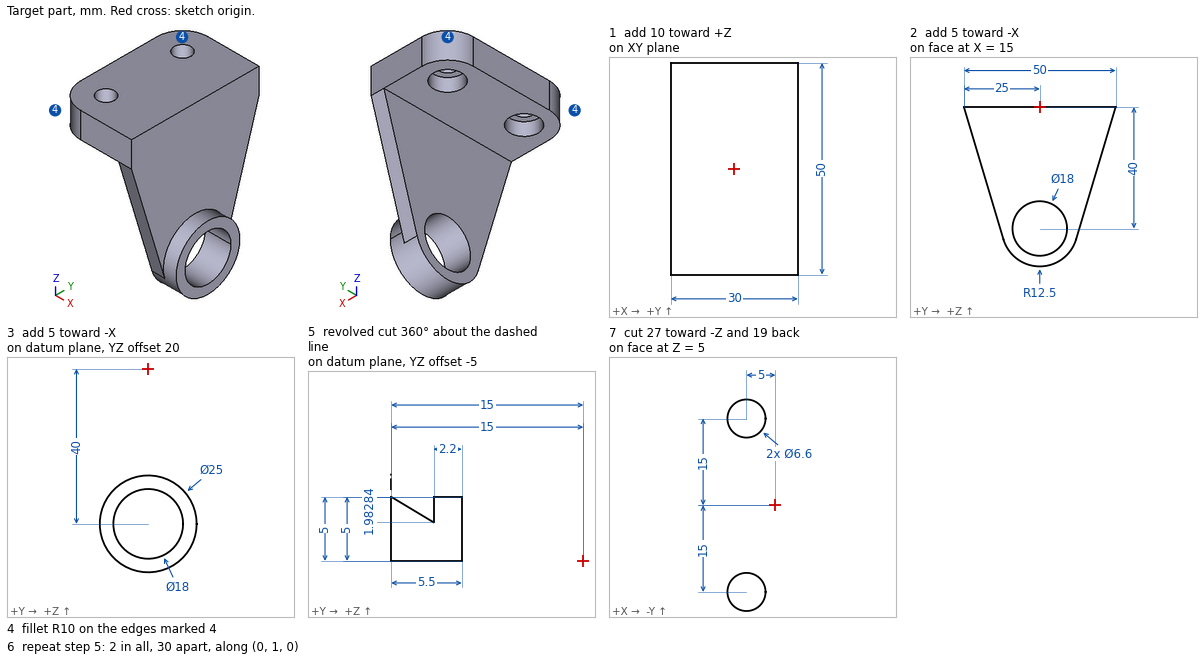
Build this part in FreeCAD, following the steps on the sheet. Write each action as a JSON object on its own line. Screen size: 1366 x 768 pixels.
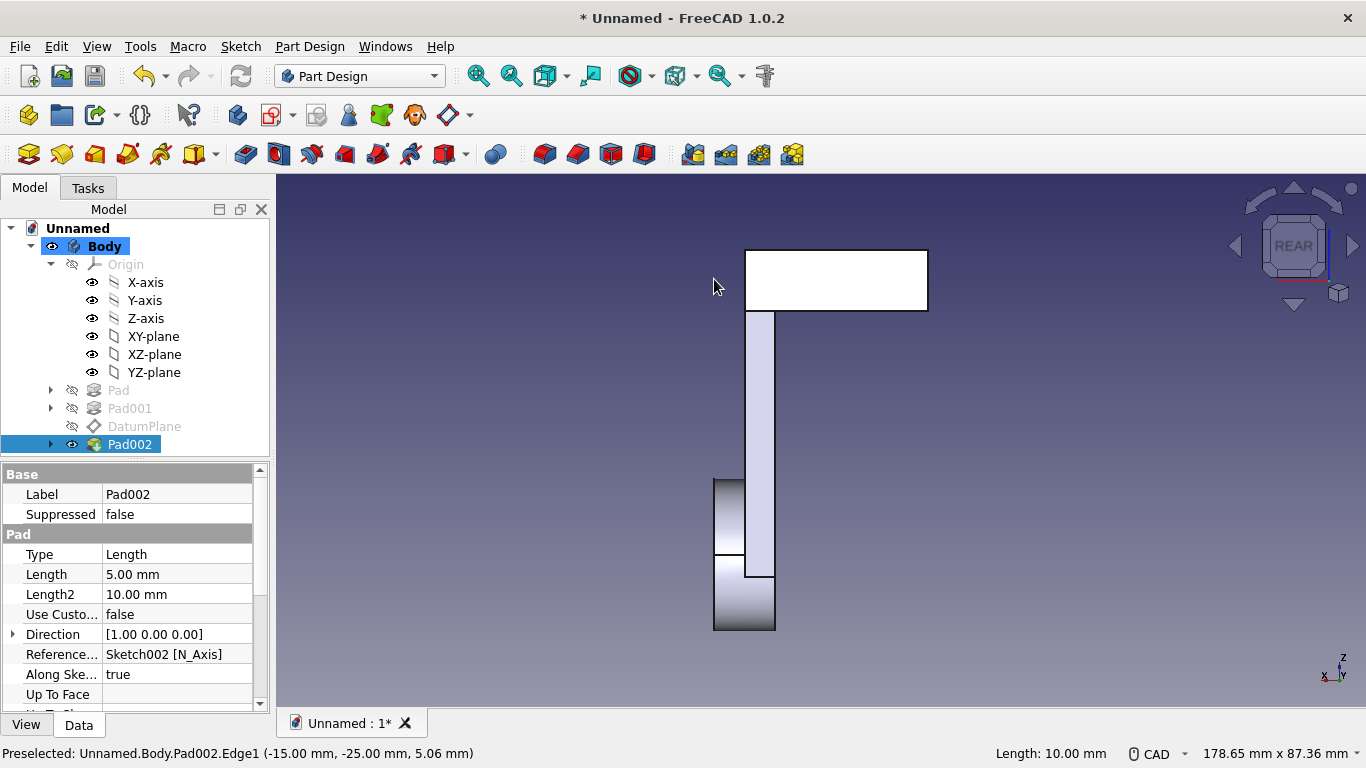
{"action": "left_click", "coordinate": [928, 279], "text": "ctrl"}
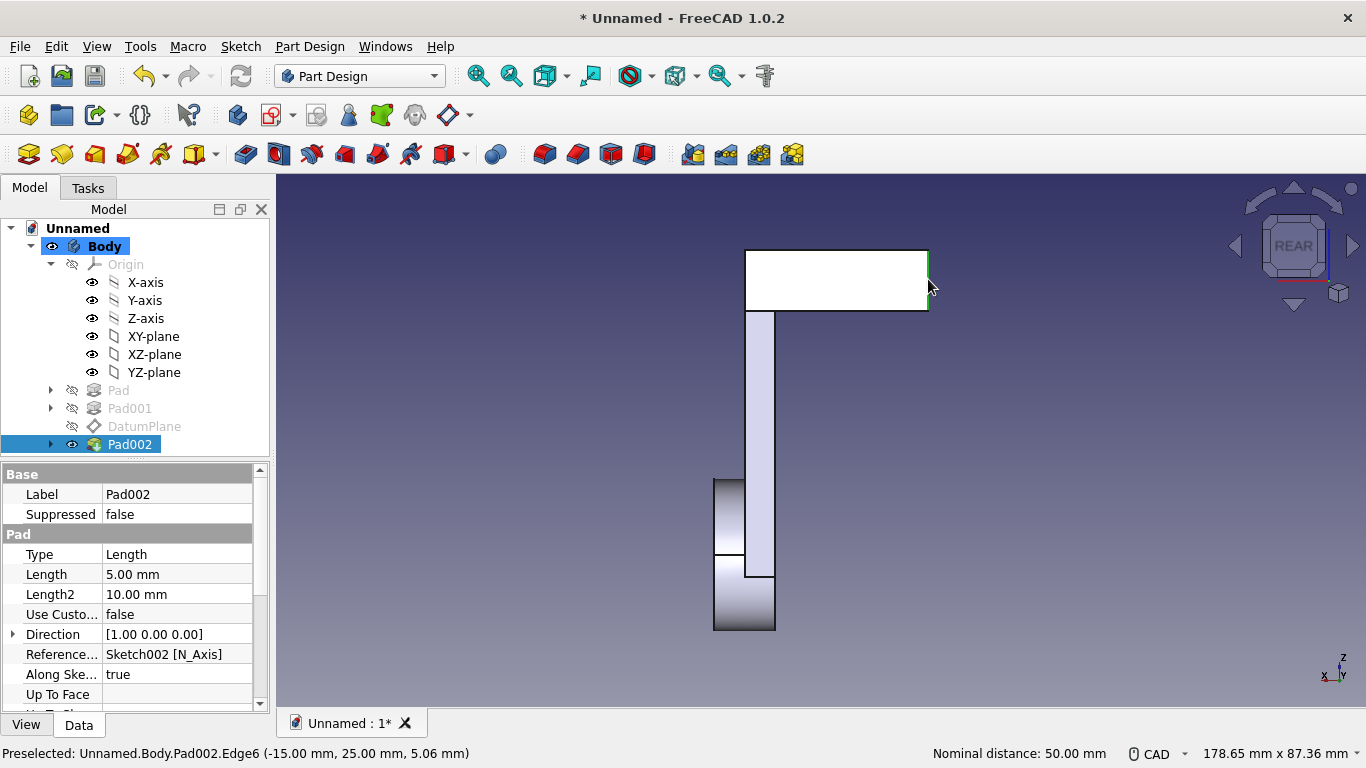
{"action": "left_click", "coordinate": [545, 154]}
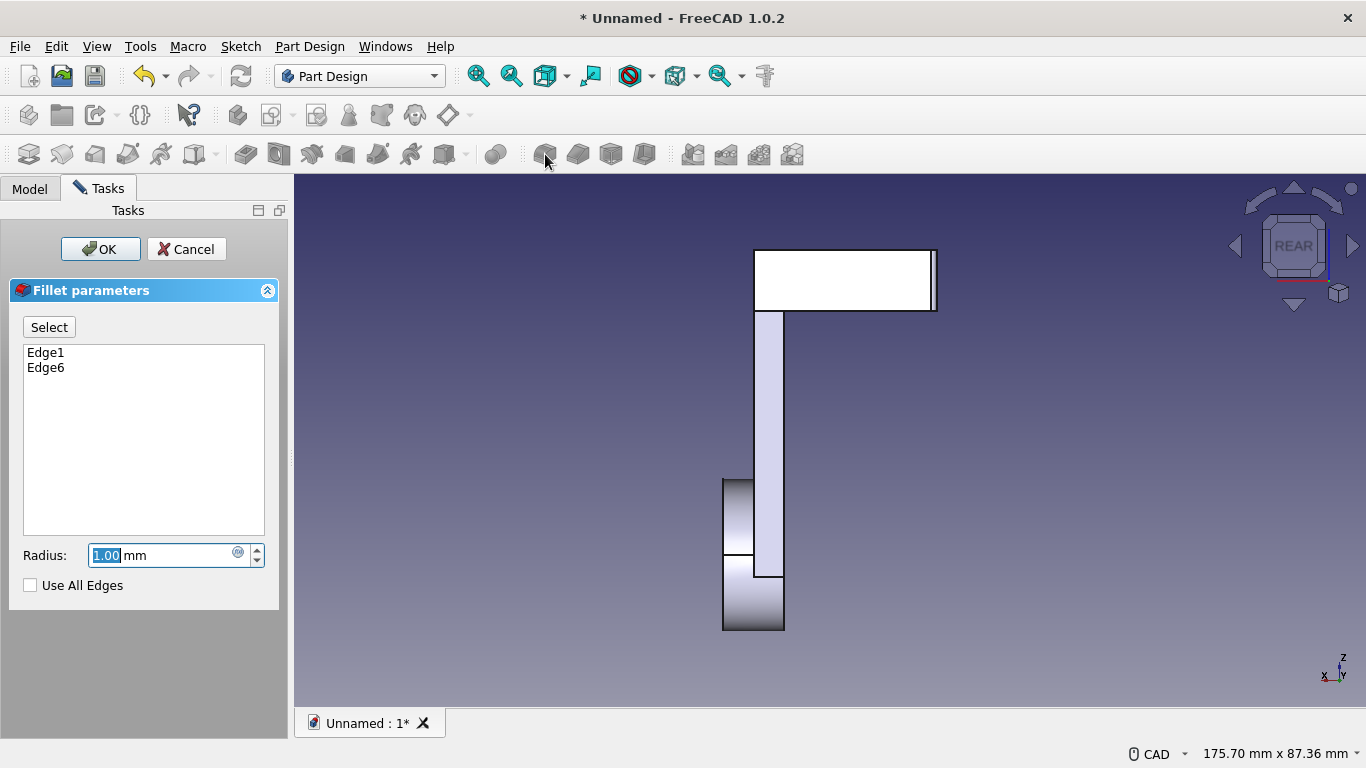
{"action": "type", "text": "10"}
{"action": "key", "text": "Tab"}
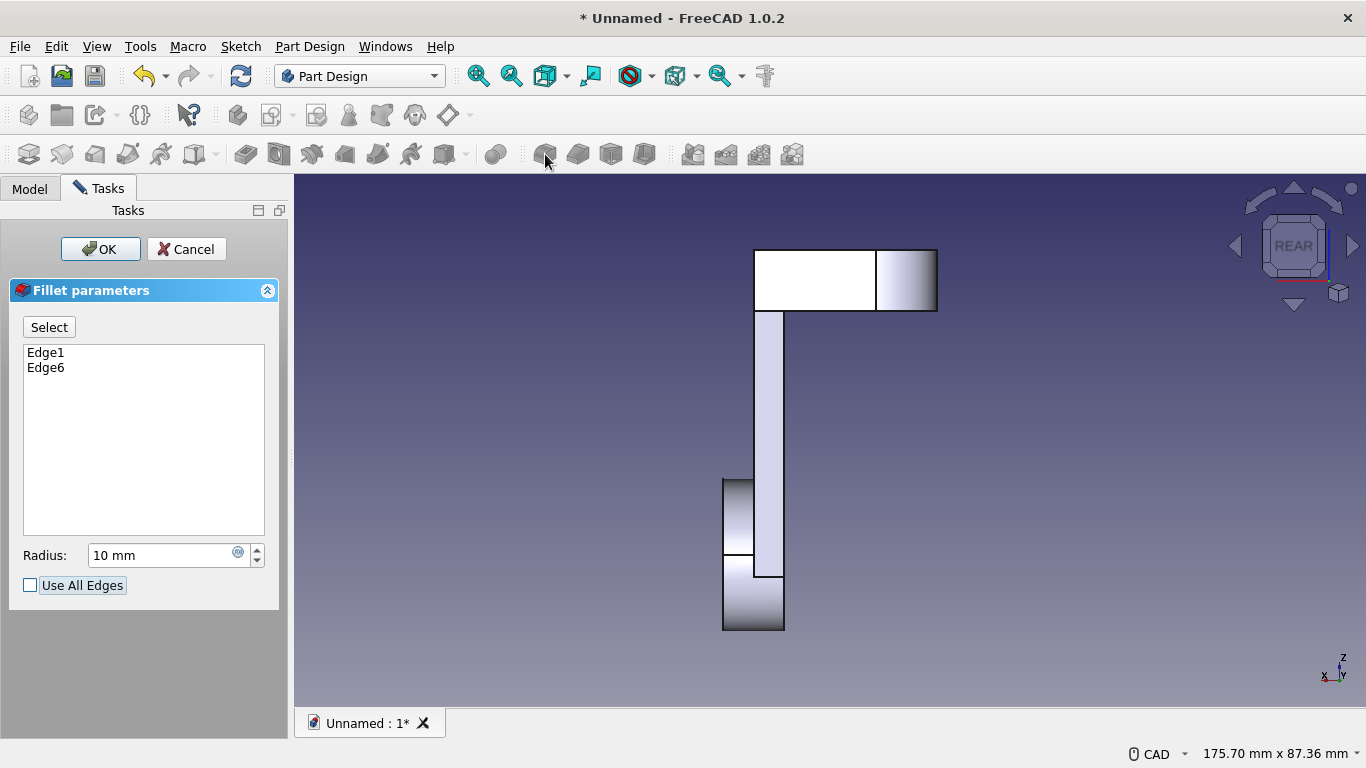
{"action": "left_click", "coordinate": [101, 249]}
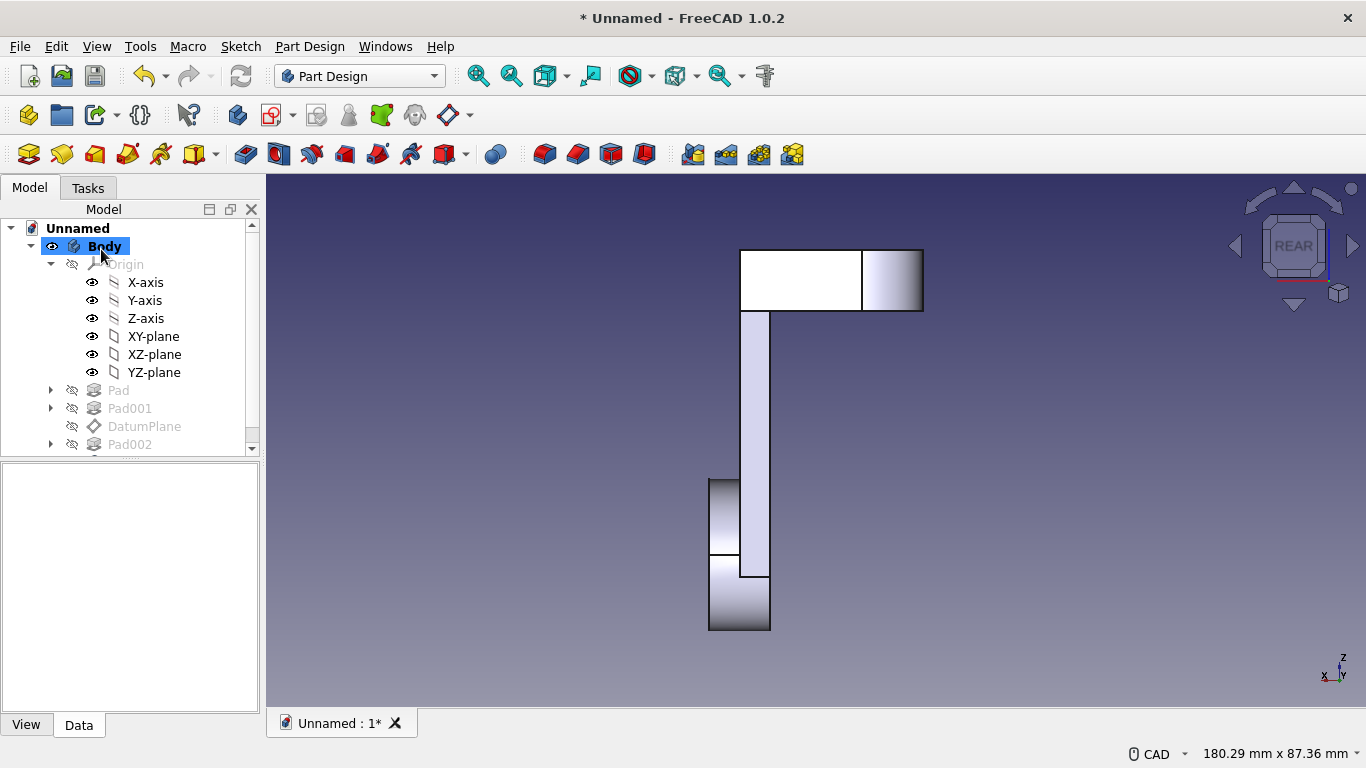
{"action": "left_click", "coordinate": [137, 372]}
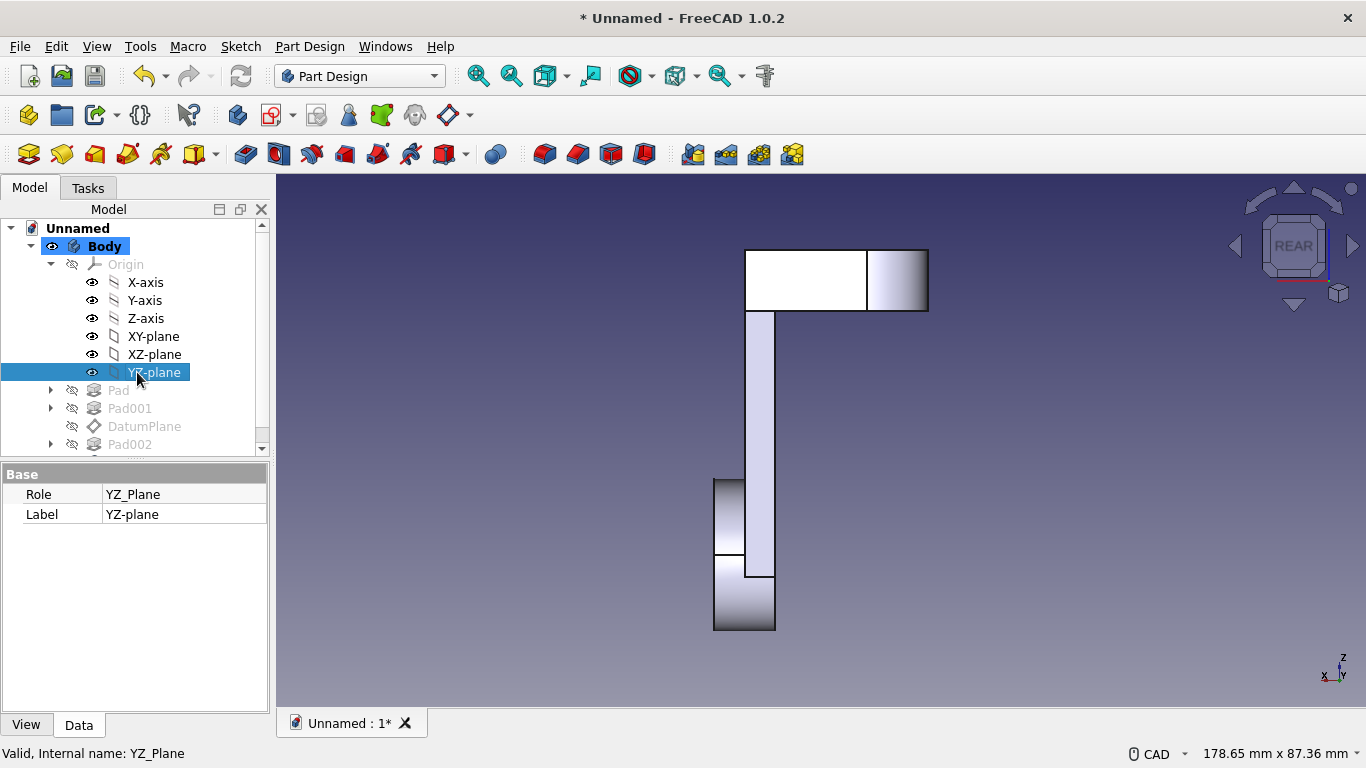
{"action": "left_click", "coordinate": [448, 116]}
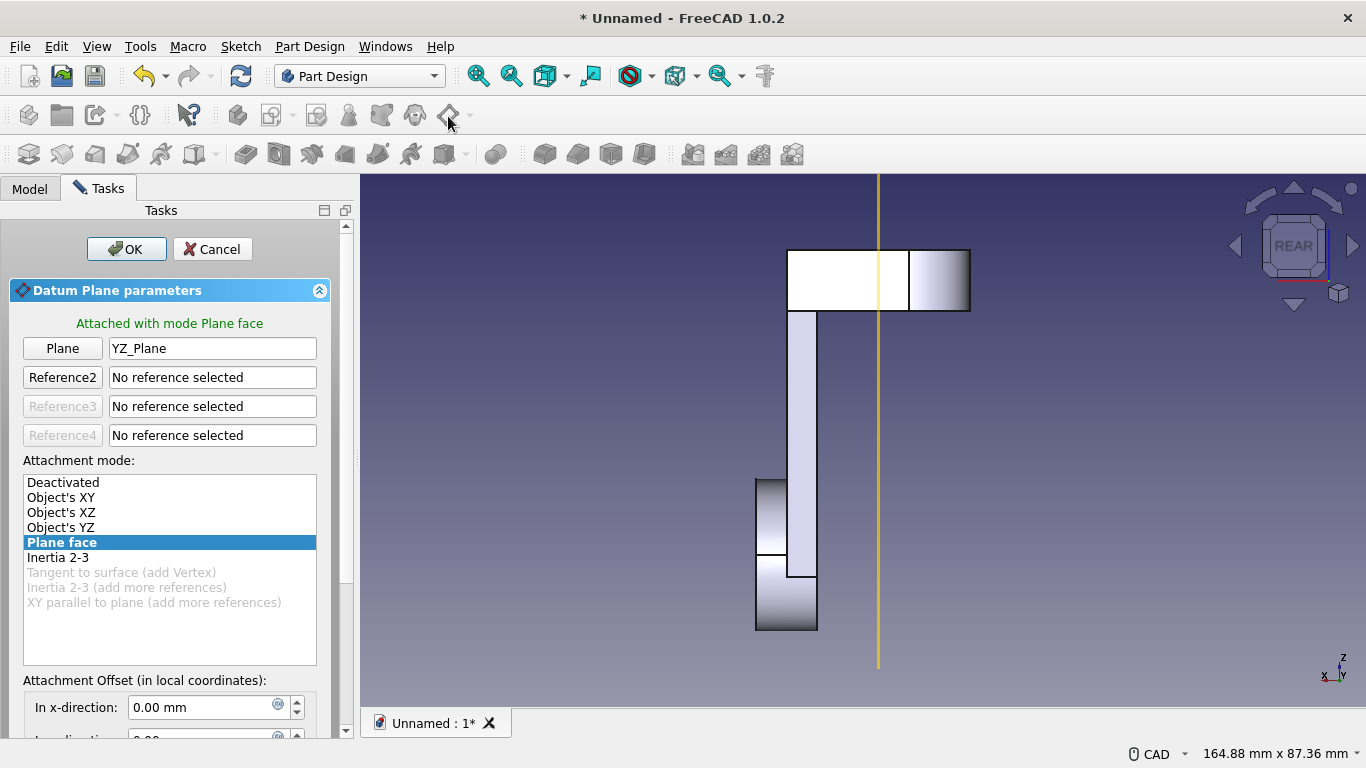
{"action": "scroll", "coordinate": [346, 479], "scroll_direction": "down", "scroll_amount": 2}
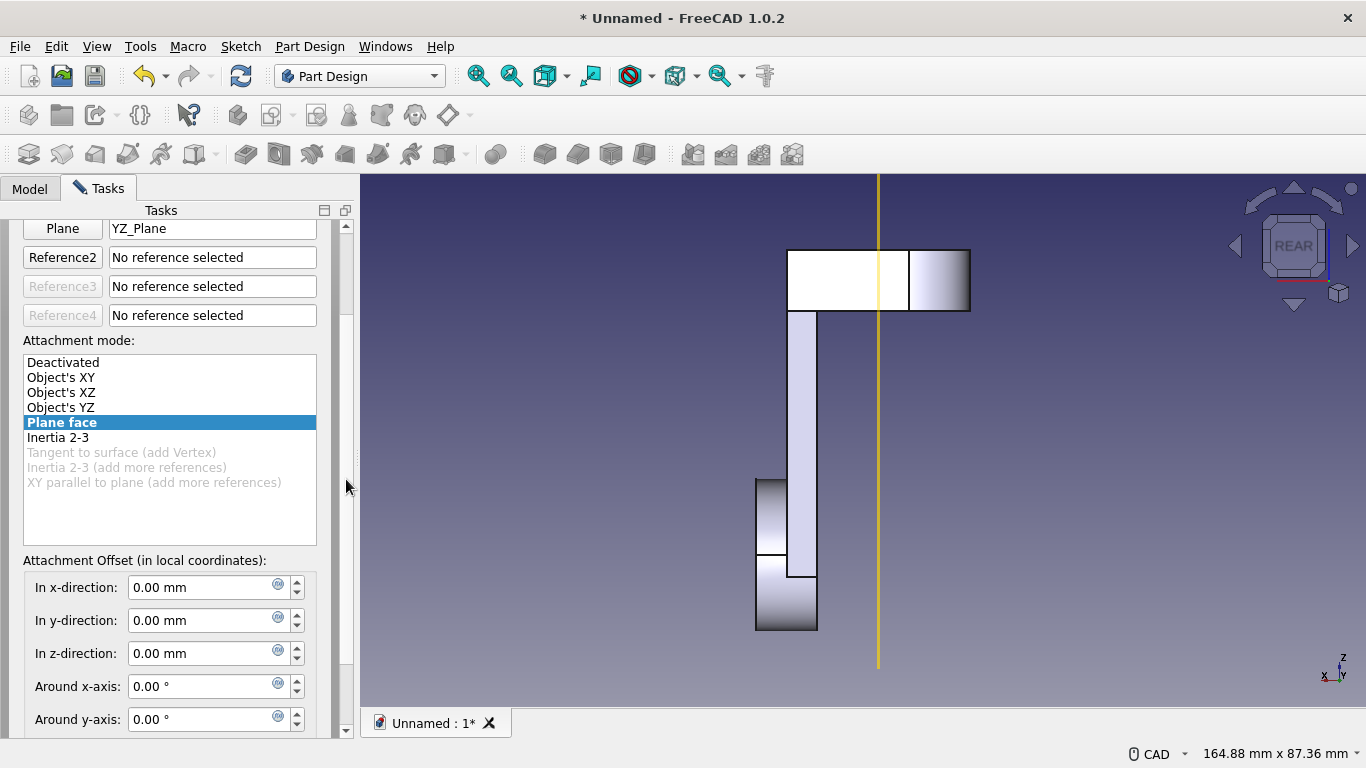
{"action": "triple_click", "coordinate": [210, 654]}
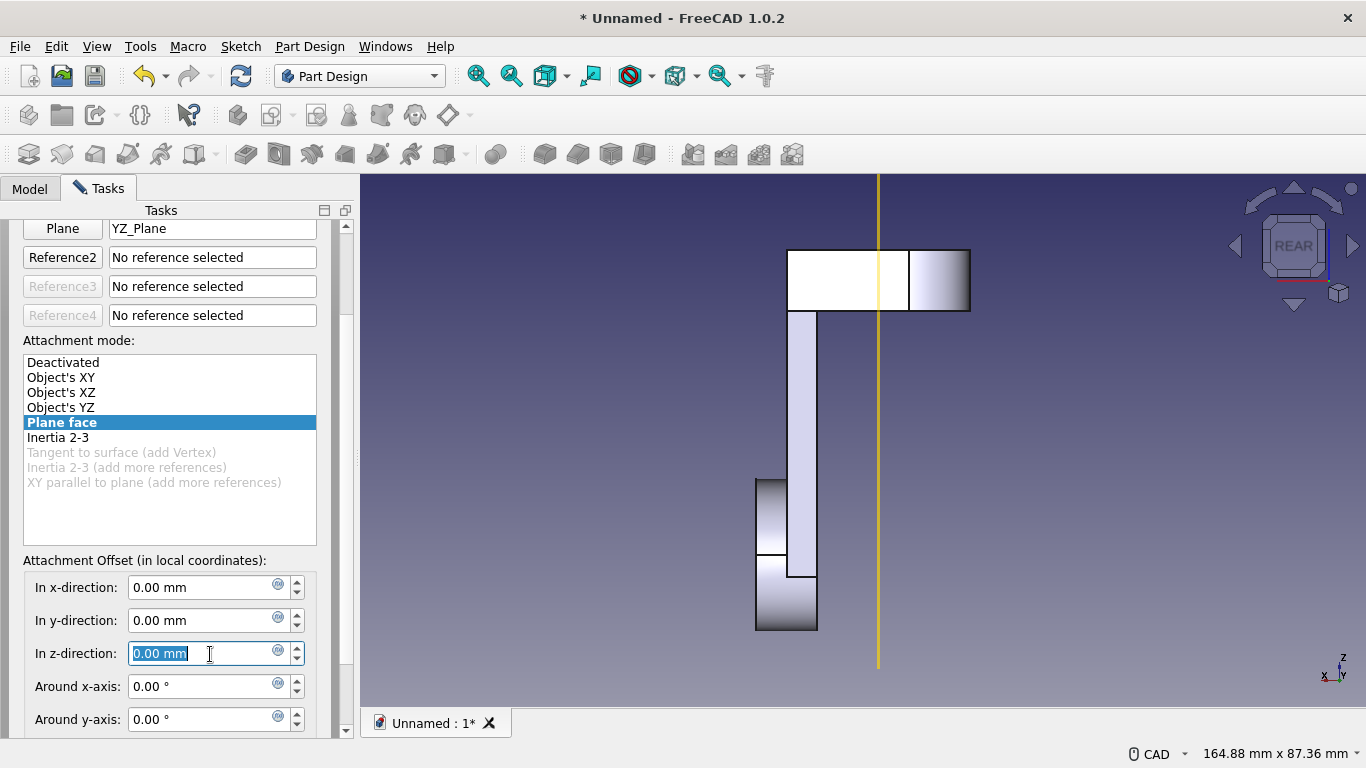
{"action": "type", "text": "-5"}
{"action": "key", "text": "Tab"}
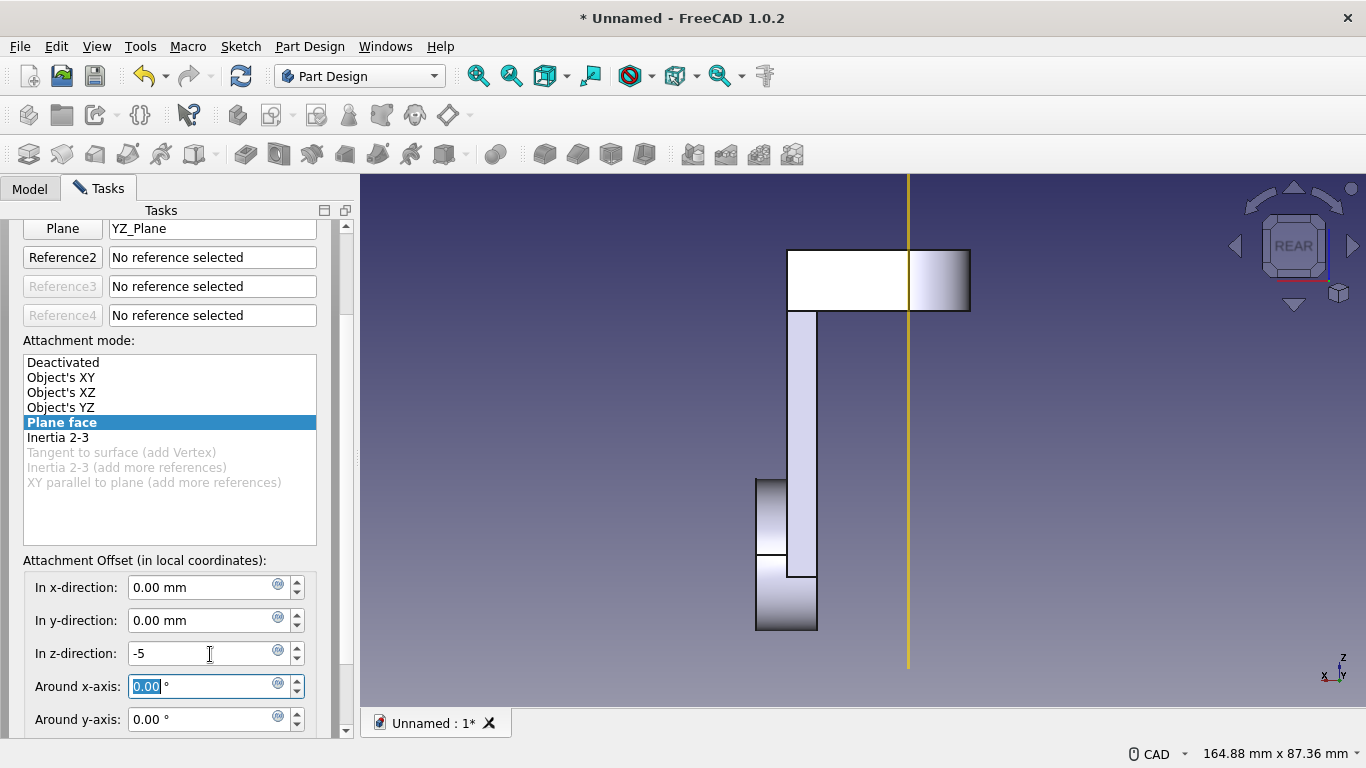
{"action": "scroll", "coordinate": [346, 479], "scroll_direction": "up", "scroll_amount": 3}